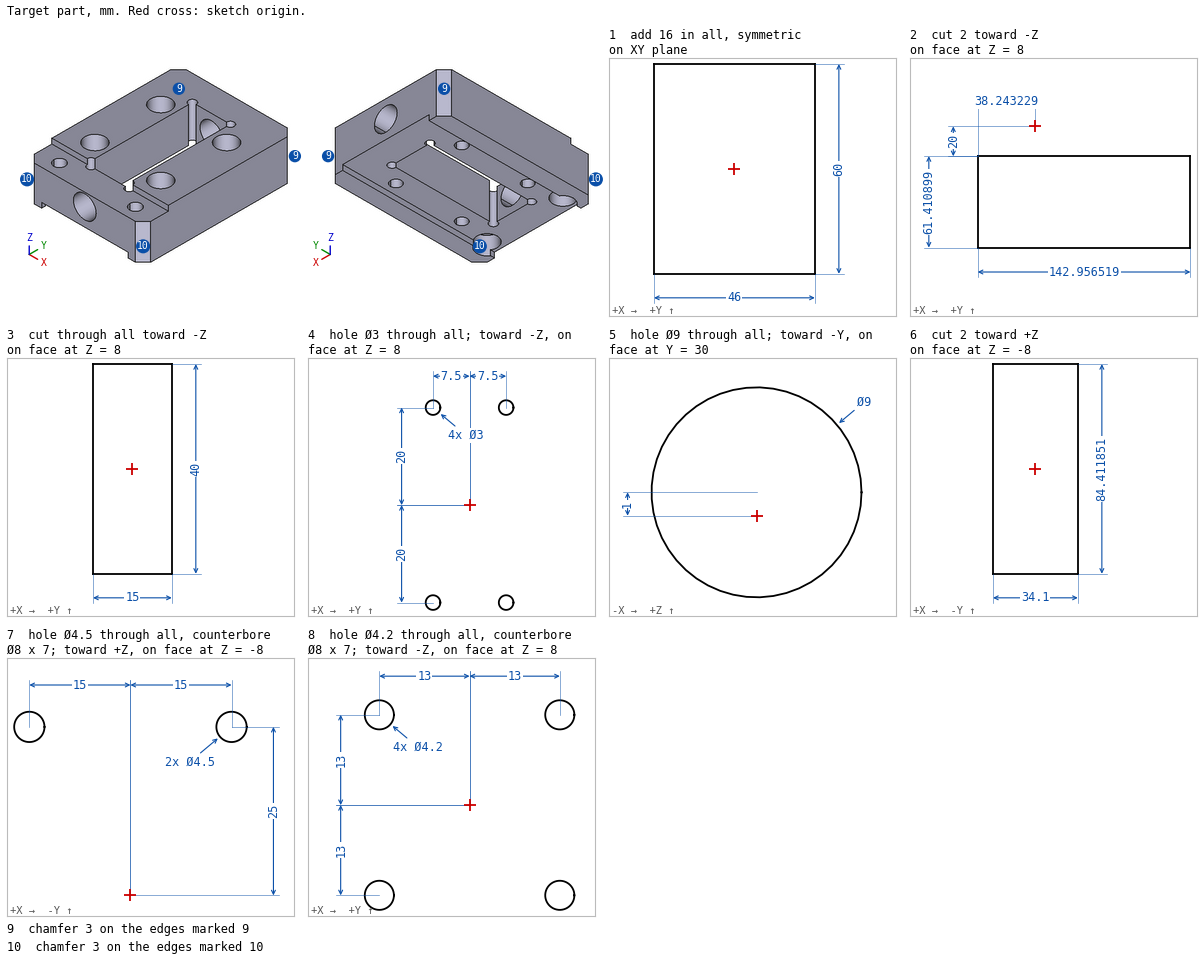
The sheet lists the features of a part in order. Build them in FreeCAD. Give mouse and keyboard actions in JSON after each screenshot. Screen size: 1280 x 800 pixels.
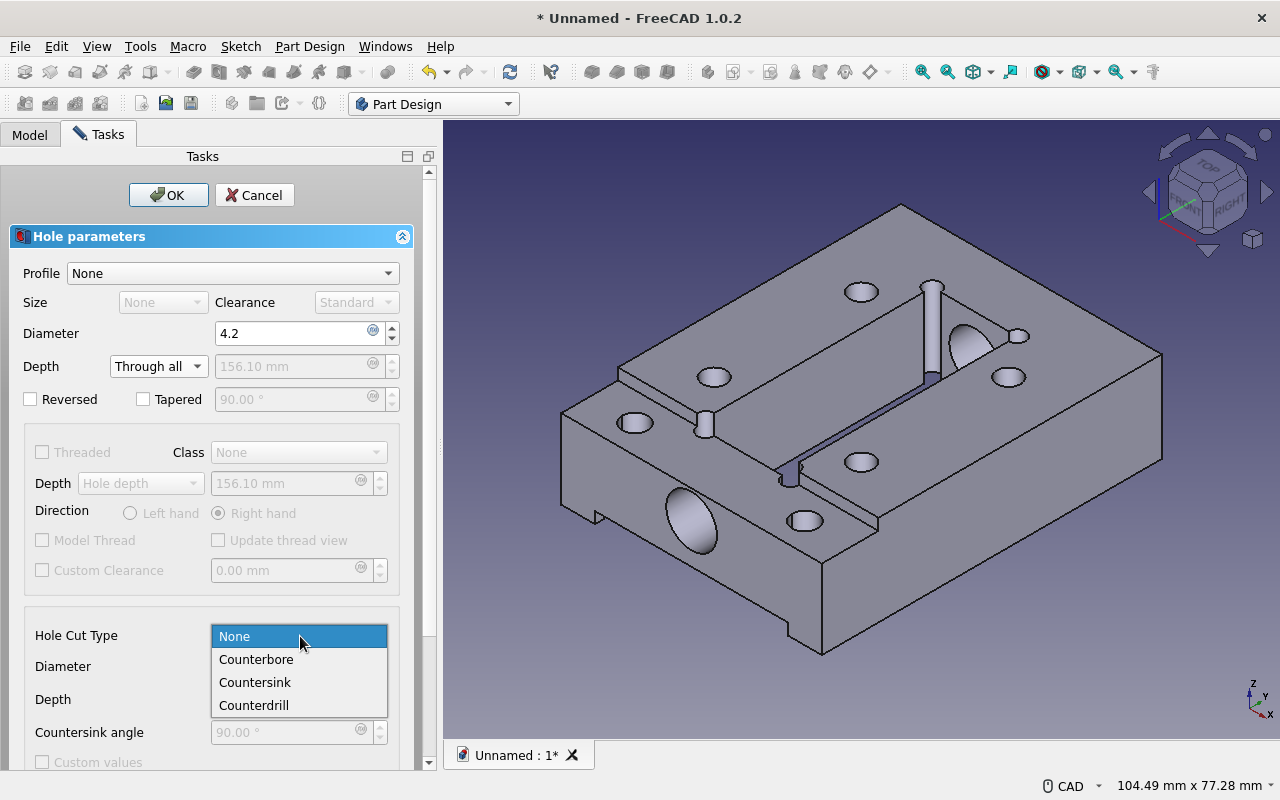
{"action": "left_click", "coordinate": [298, 660]}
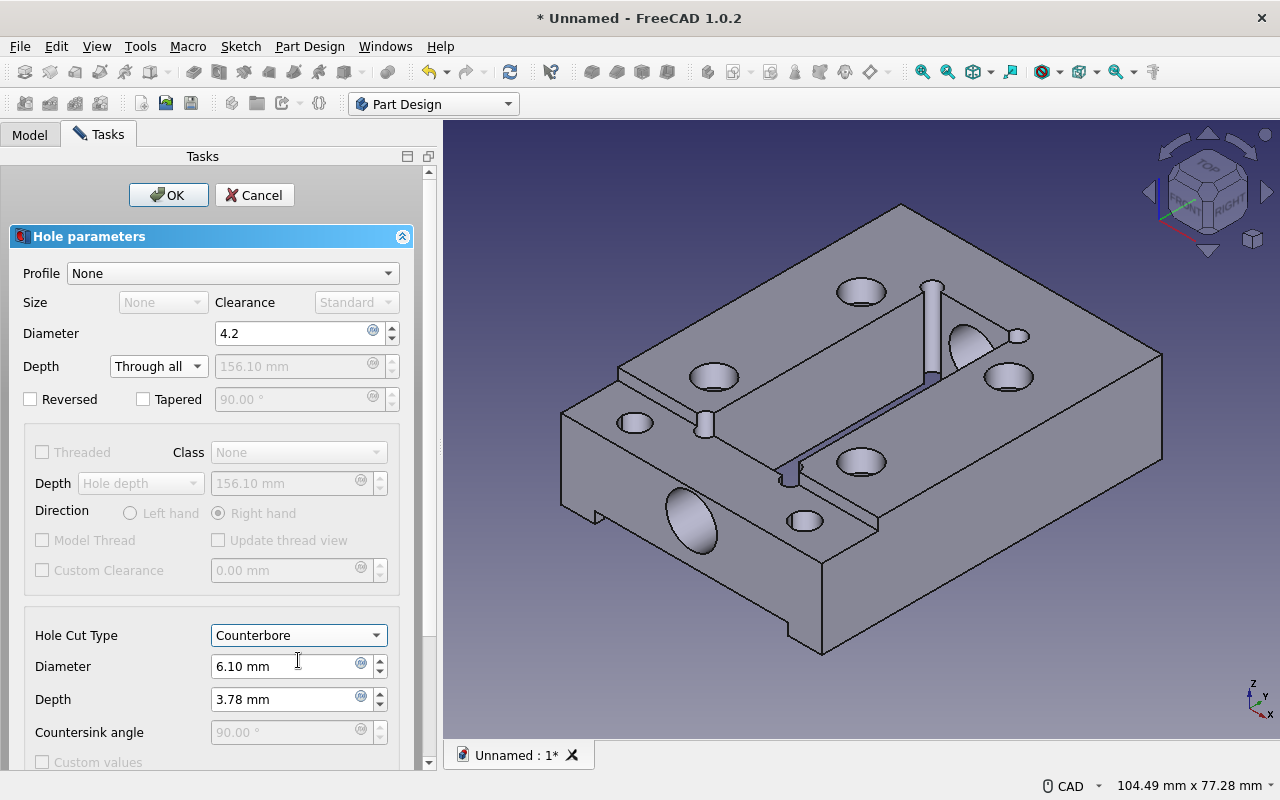
{"action": "triple_click", "coordinate": [292, 666]}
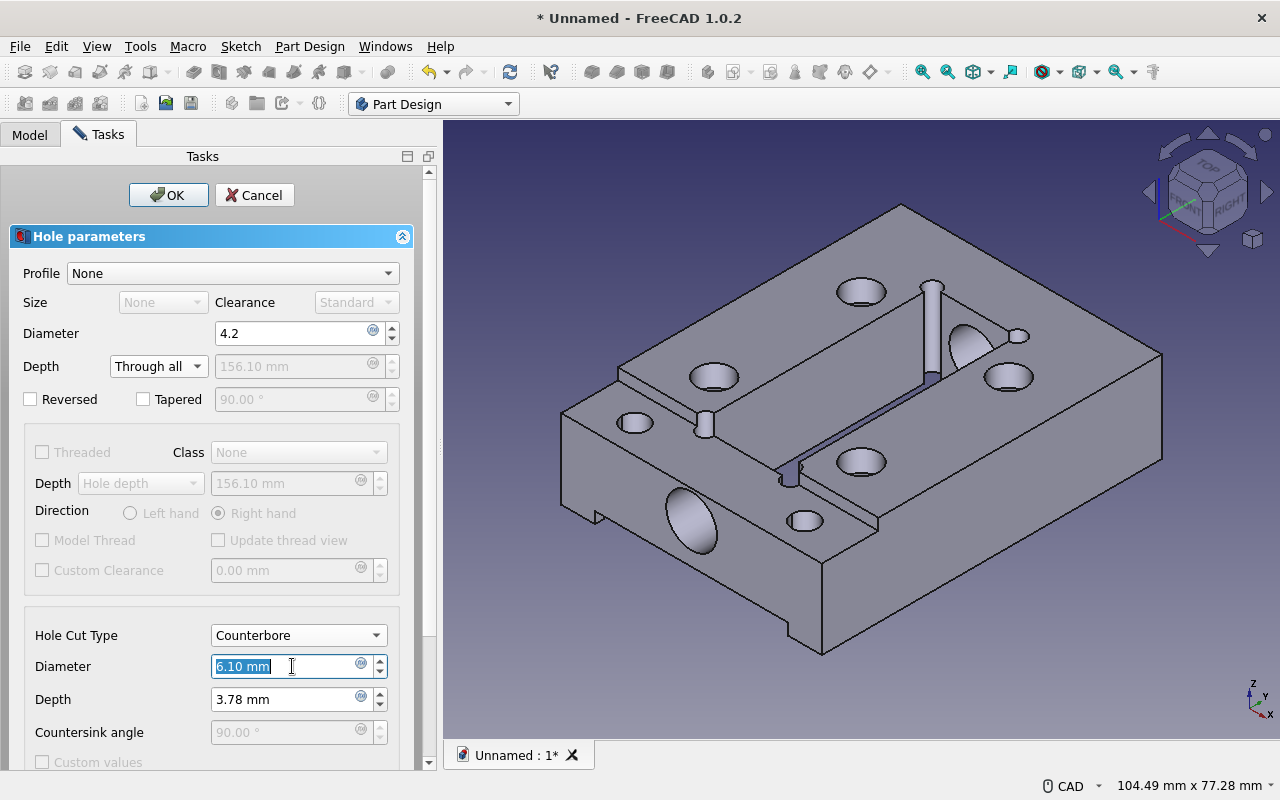
{"action": "type", "text": "8"}
{"action": "key", "text": "Tab"}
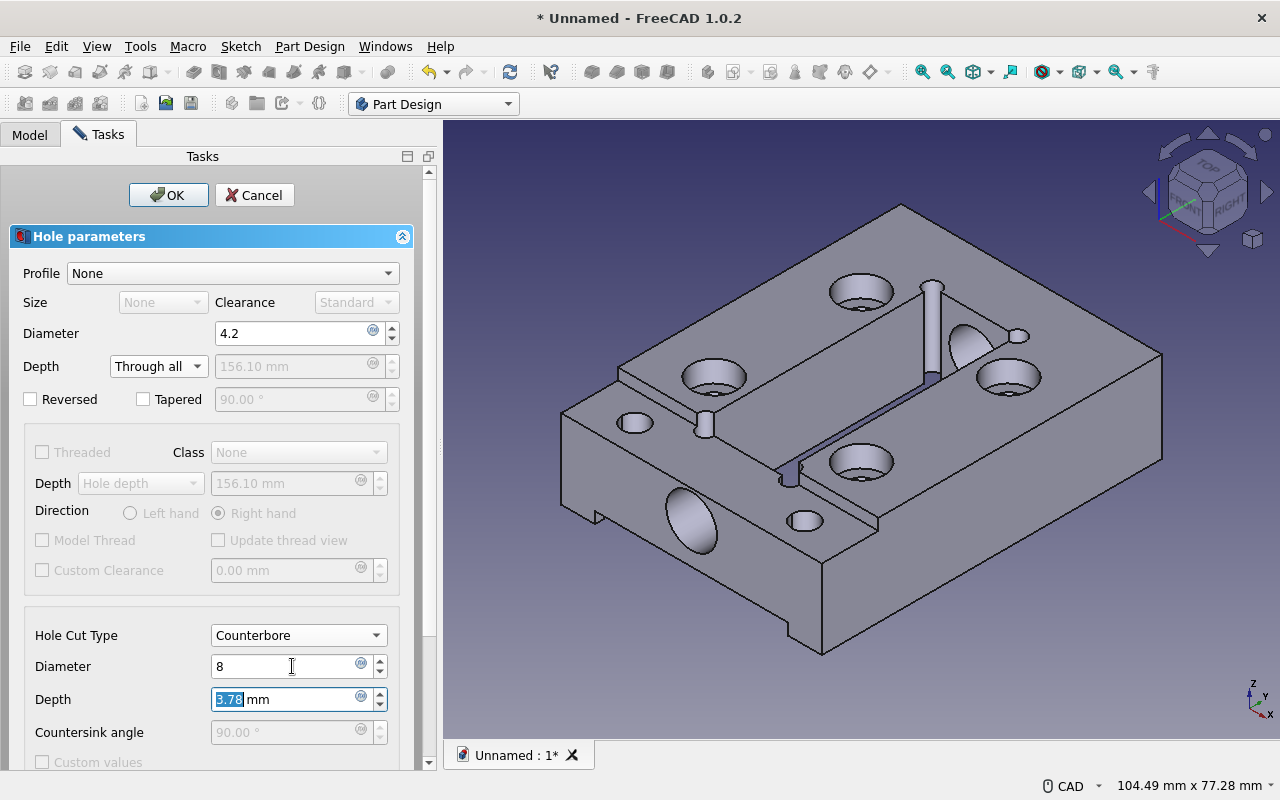
{"action": "type", "text": "7"}
{"action": "key", "text": "Tab"}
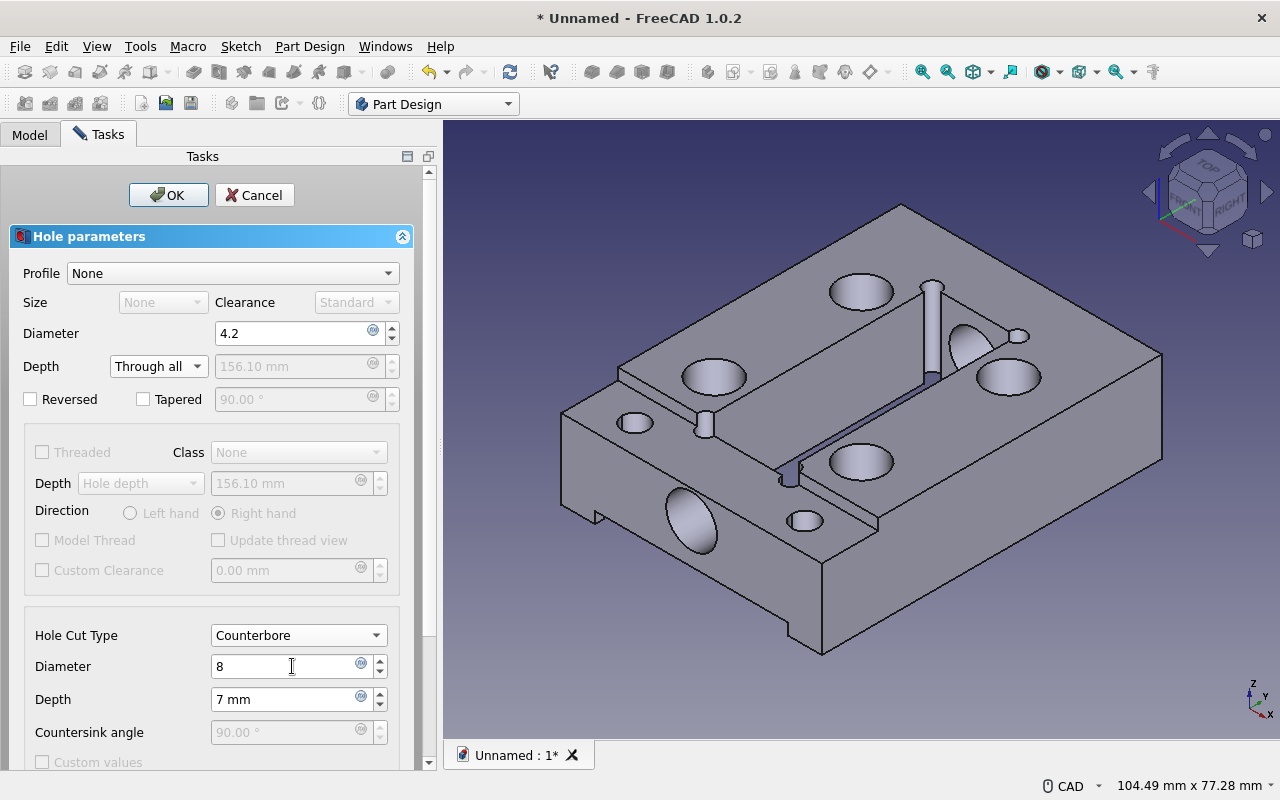
{"action": "left_click", "coordinate": [169, 195]}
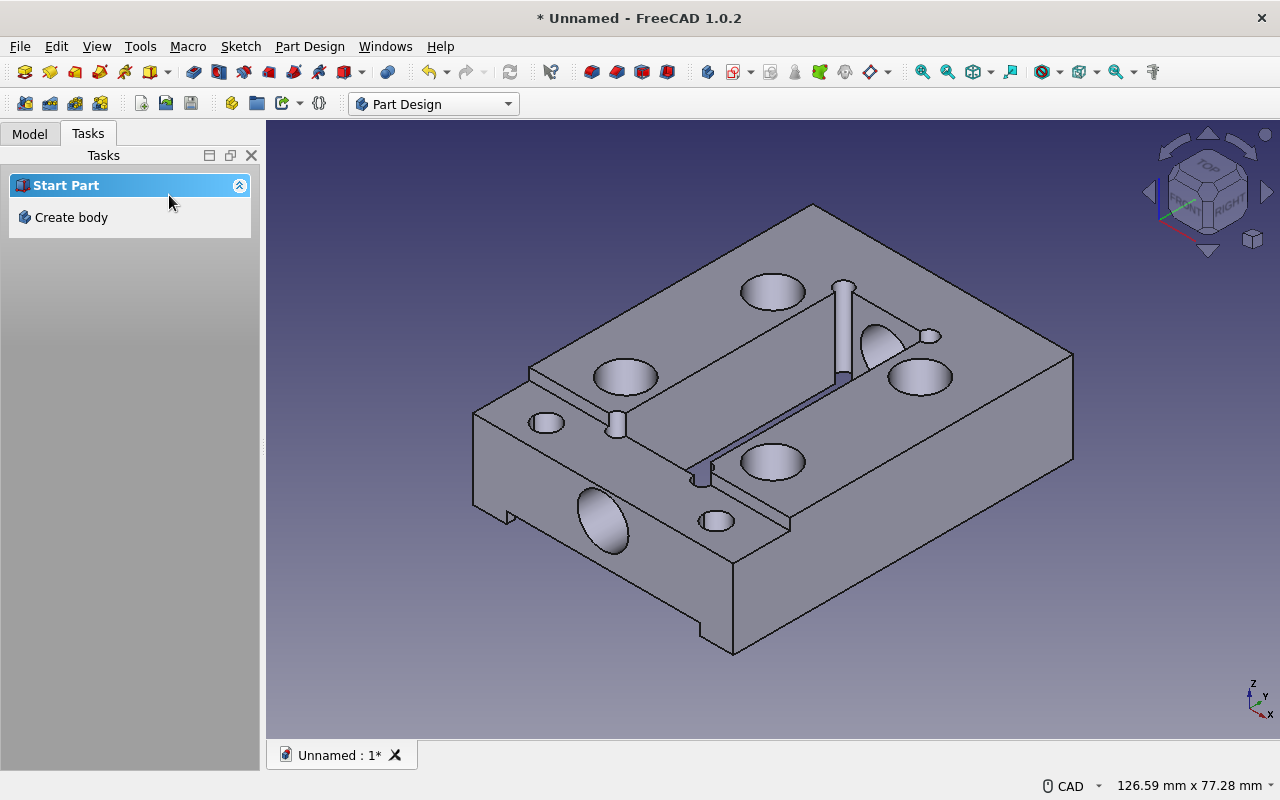
{"action": "key", "text": "2"}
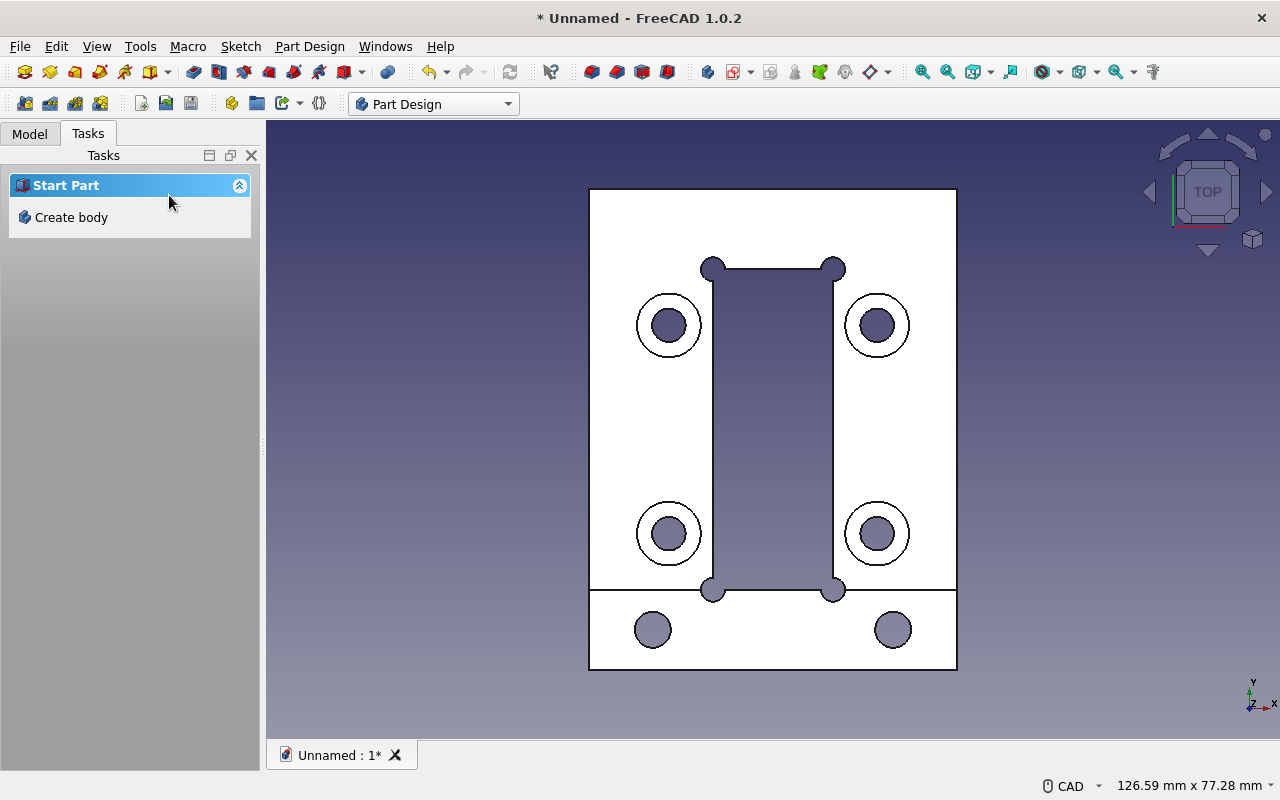
{"action": "key", "text": "0"}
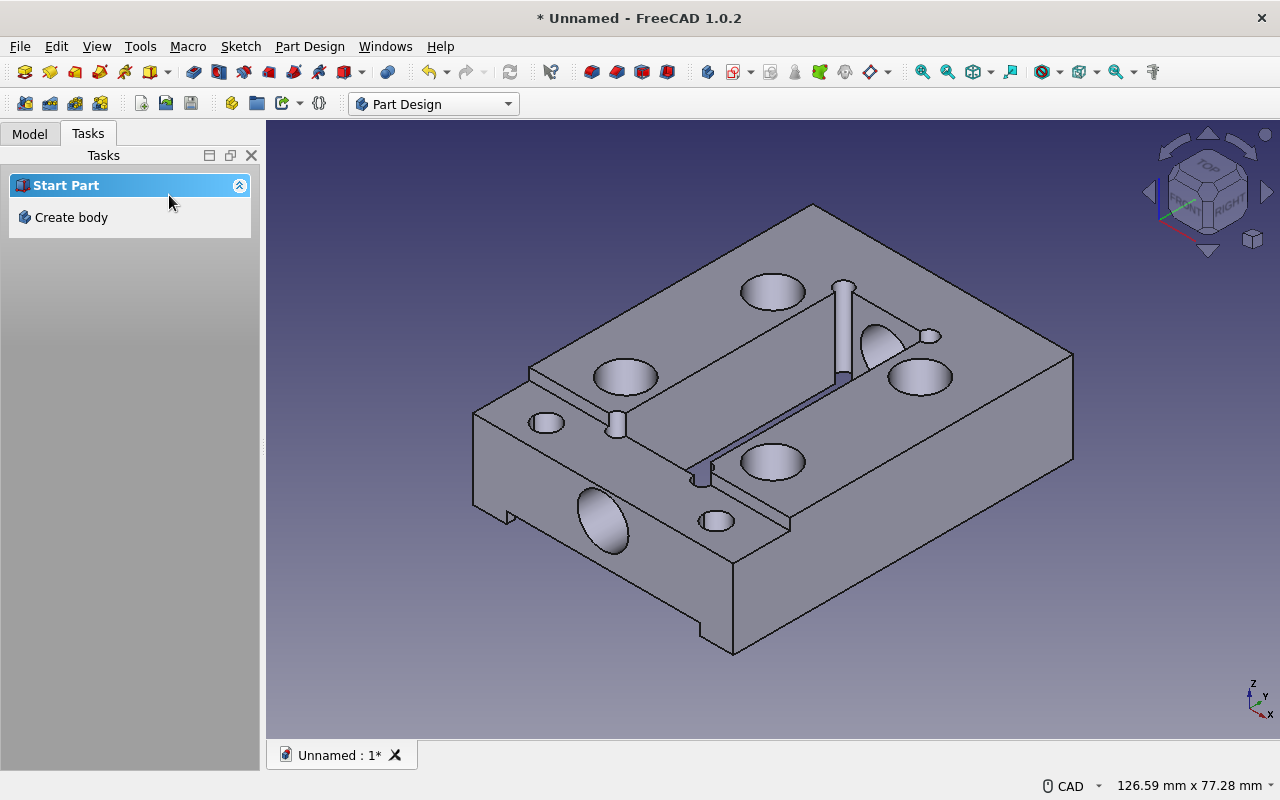
{"action": "key", "text": "1"}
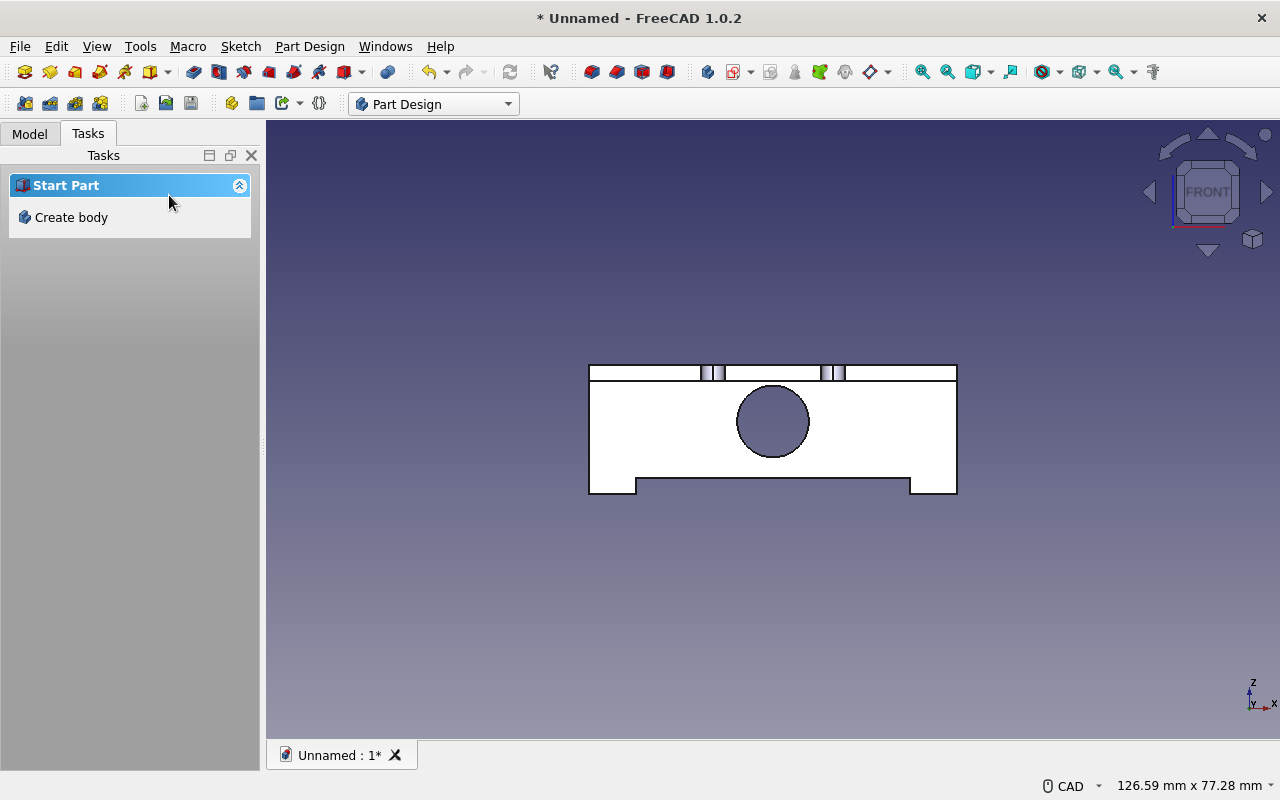
{"action": "left_click", "coordinate": [923, 72]}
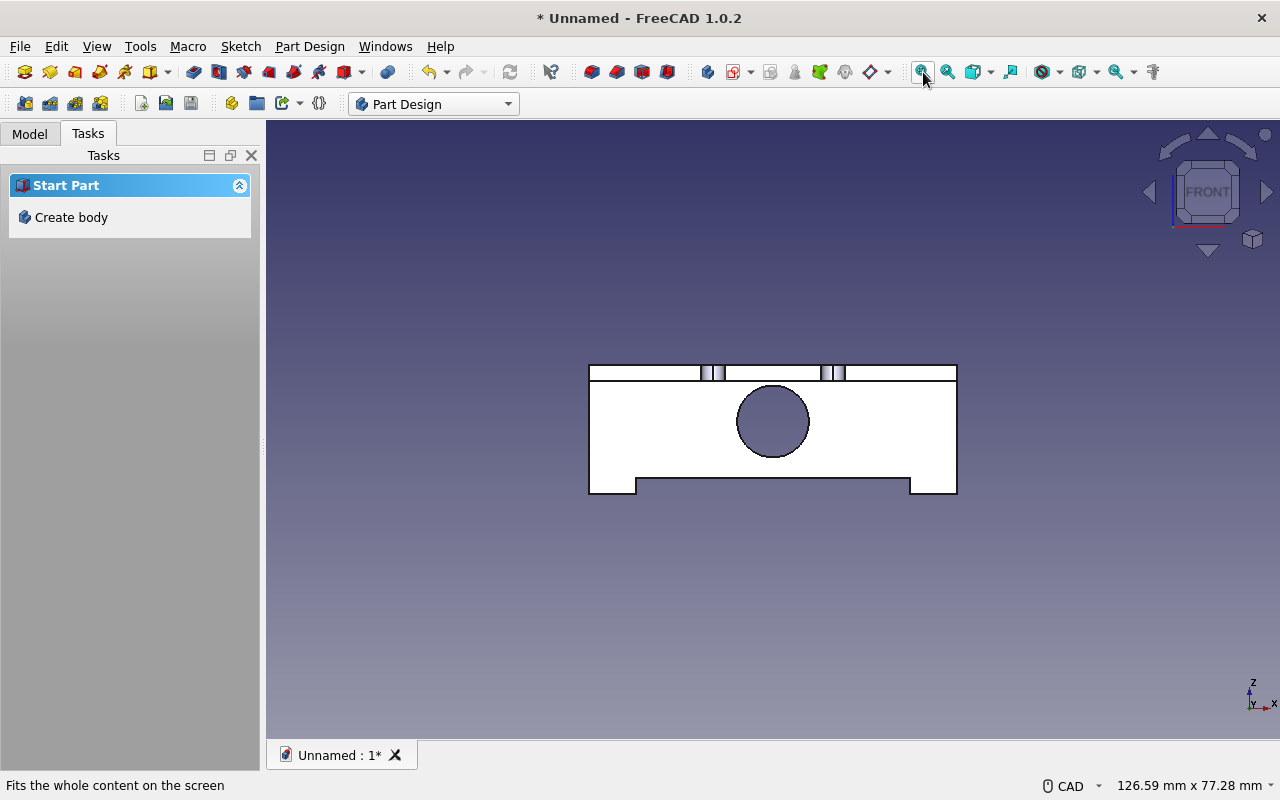
{"action": "key", "text": "3"}